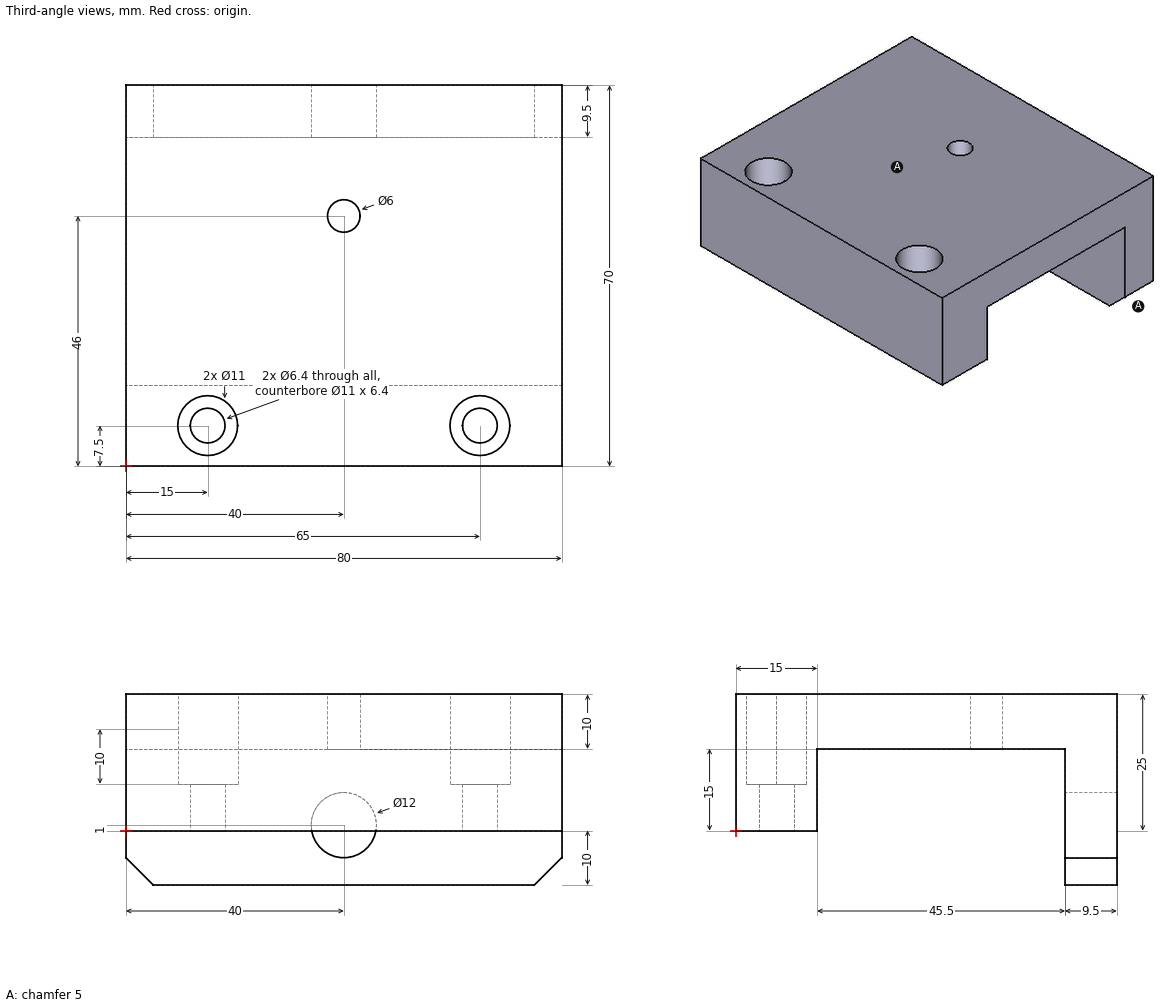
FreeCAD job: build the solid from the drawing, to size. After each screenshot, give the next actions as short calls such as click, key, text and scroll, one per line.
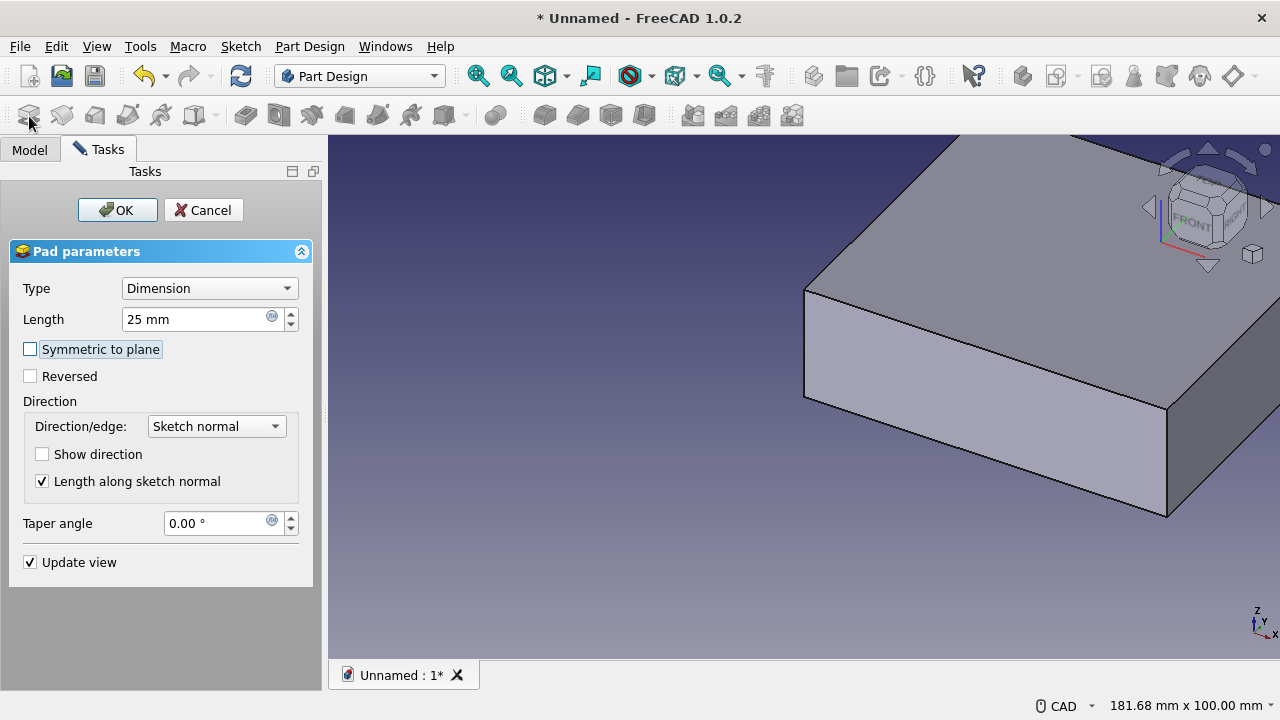
click(118, 210)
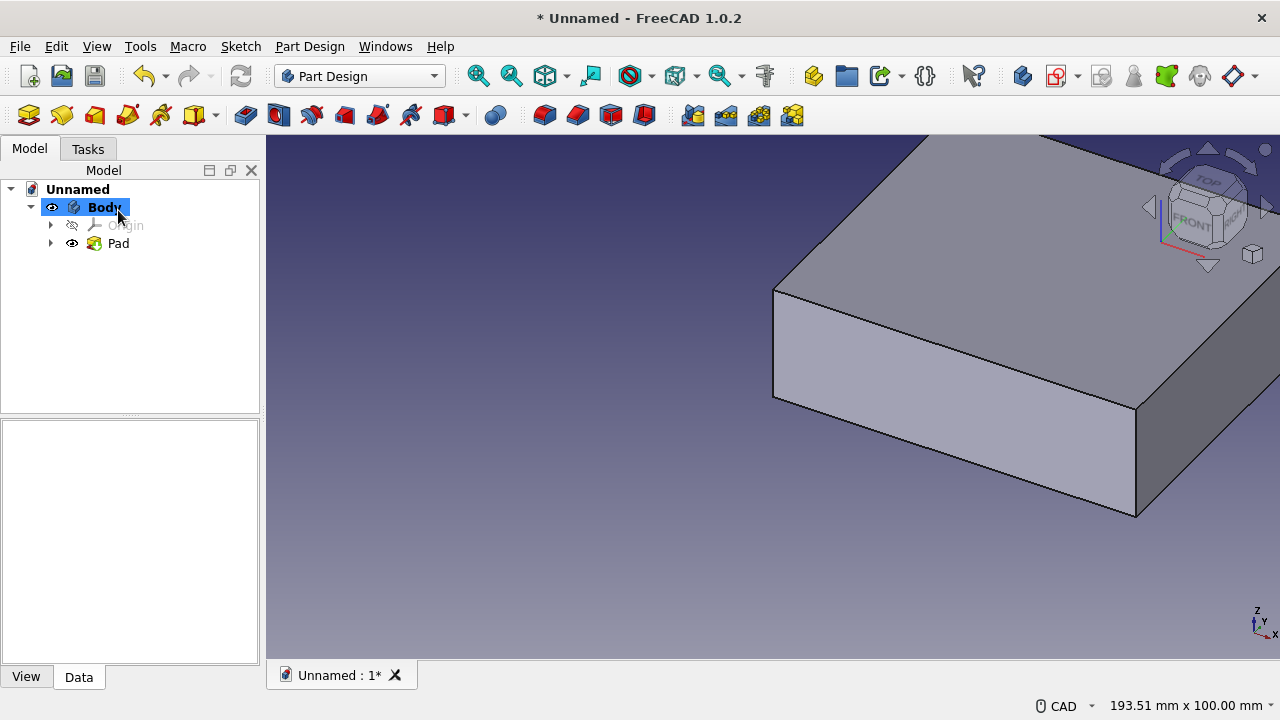
click(479, 76)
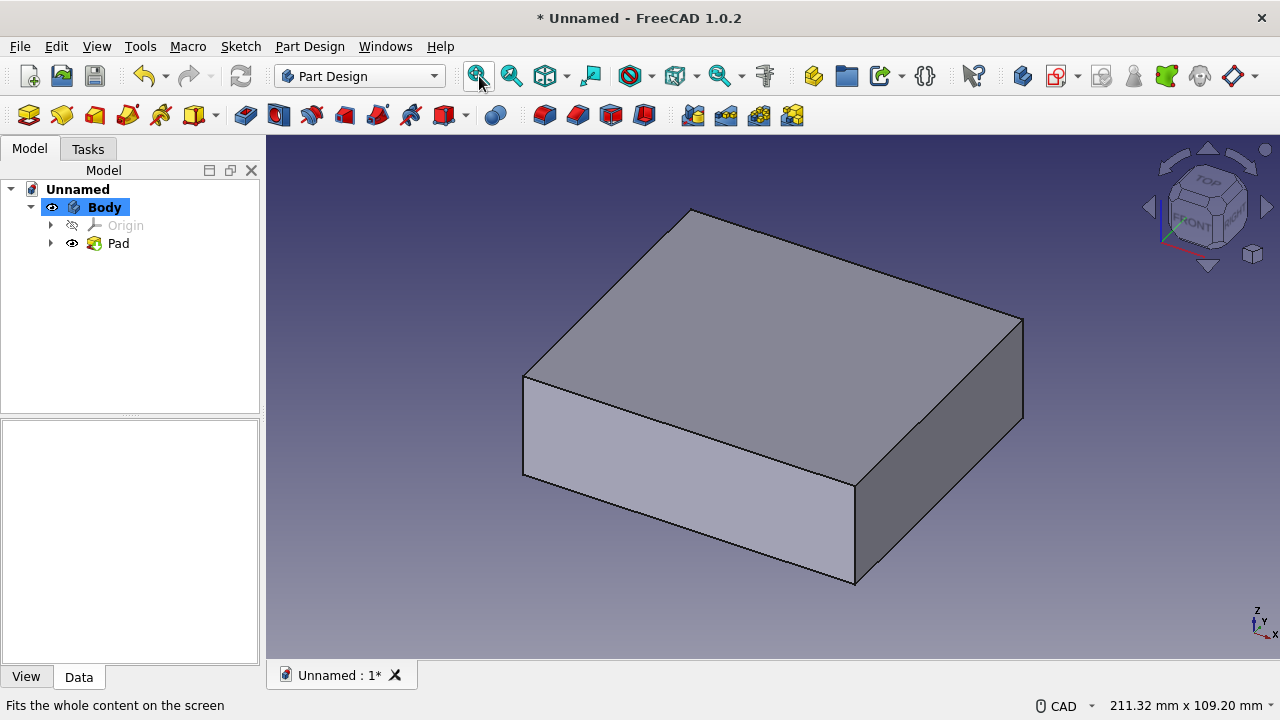
click(987, 403)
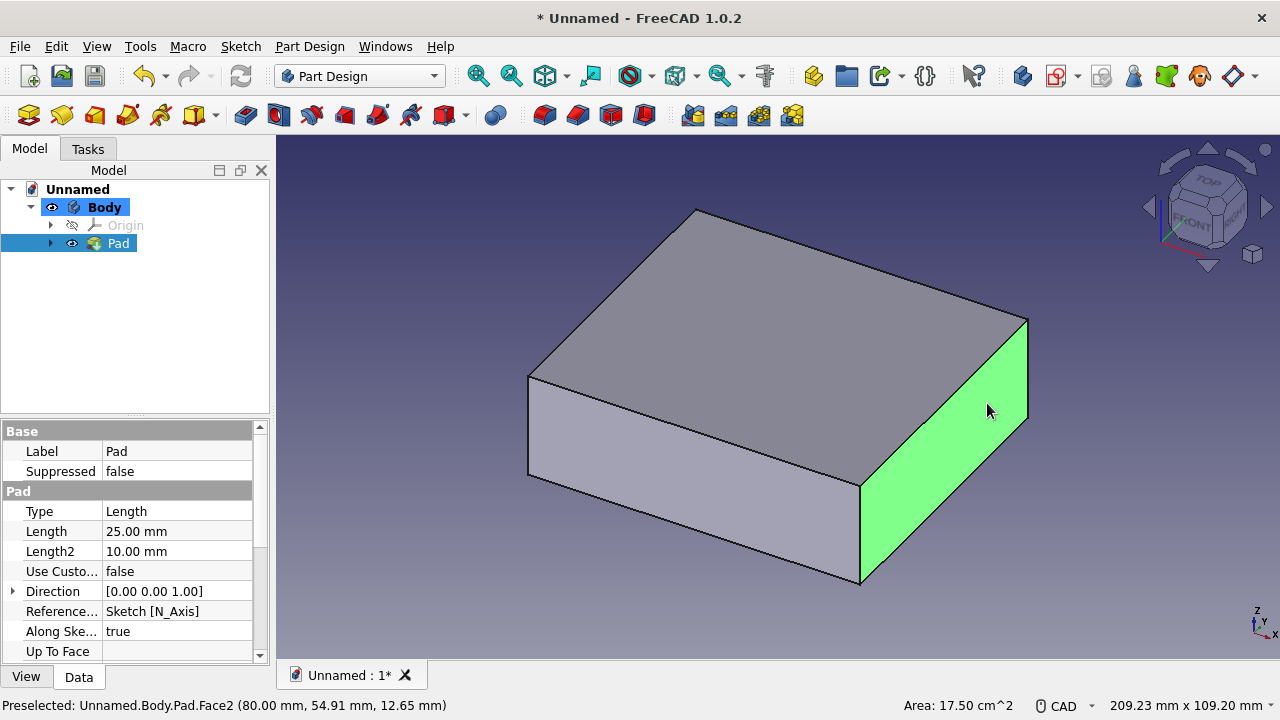
click(1056, 76)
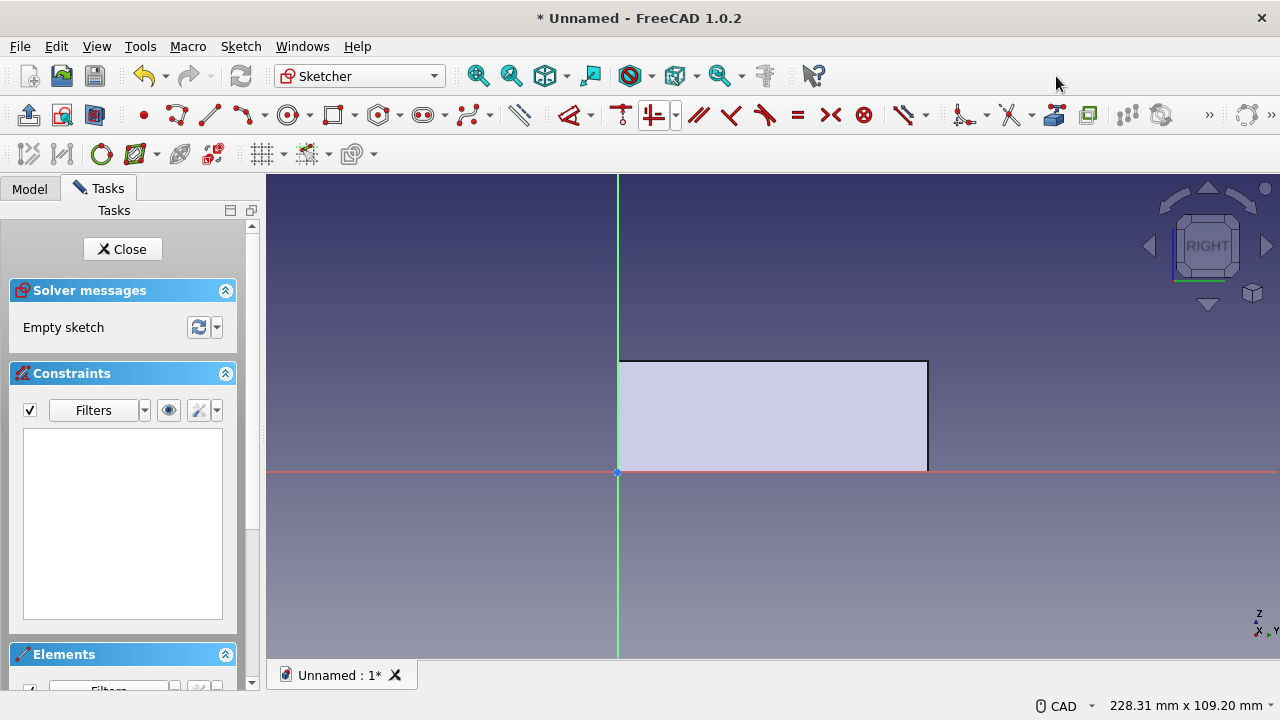
scroll(791, 457, up, 4)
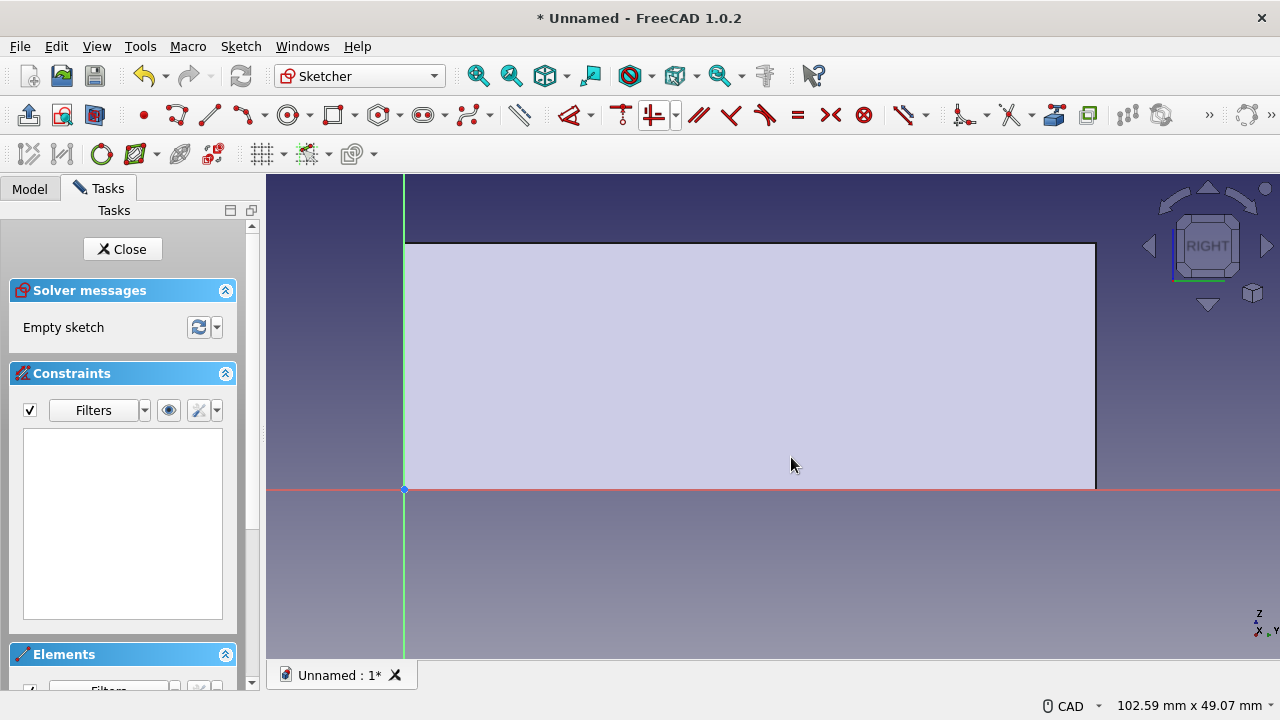
click(332, 116)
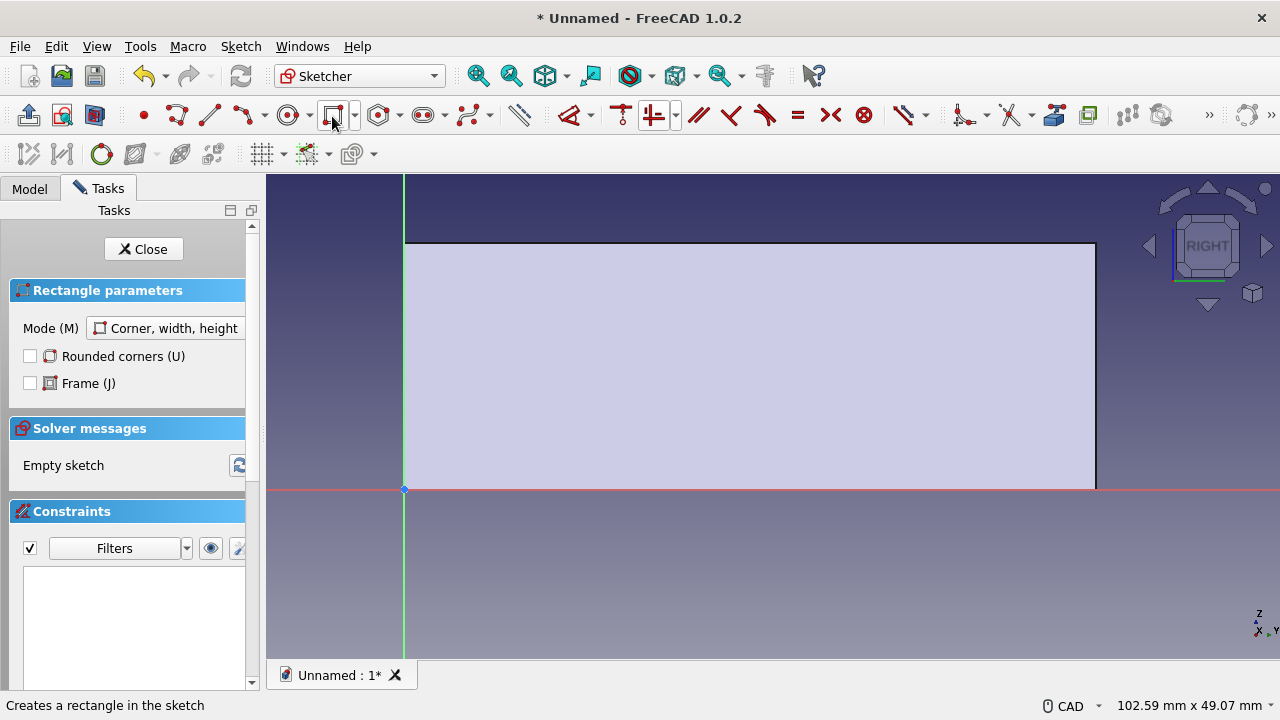
click(553, 341)
click(1002, 490)
key(Escape)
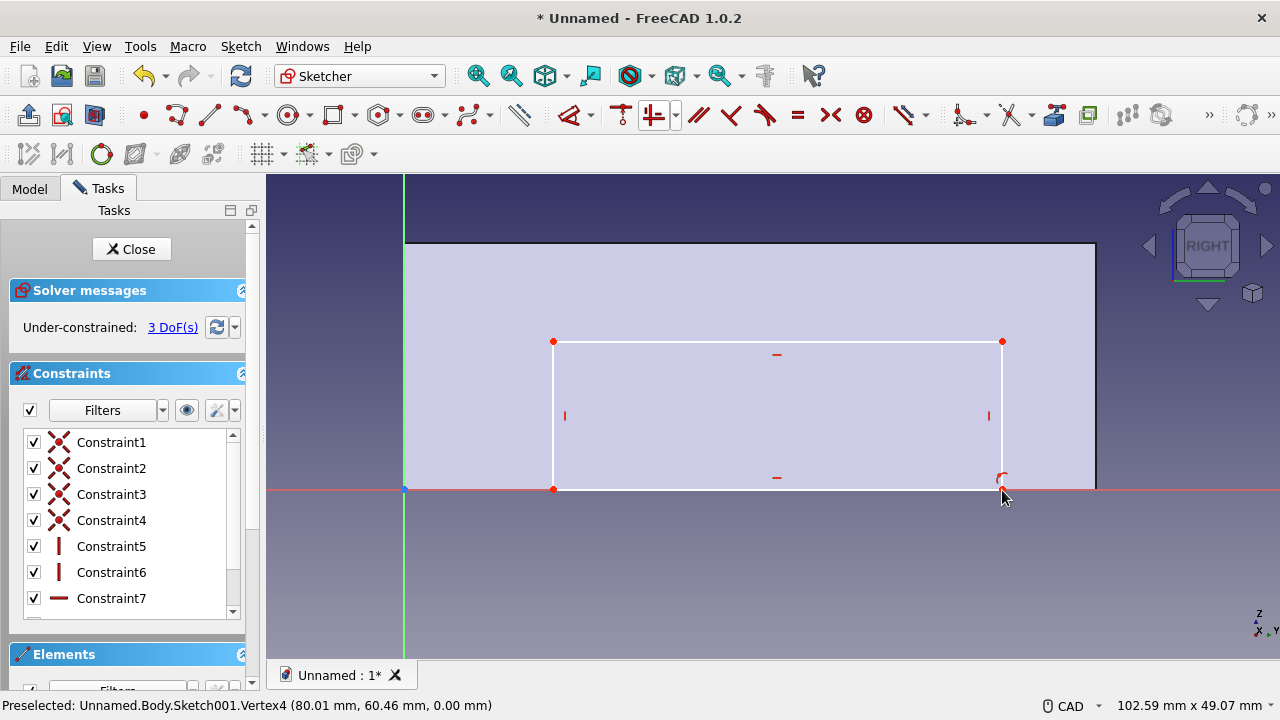
click(553, 386)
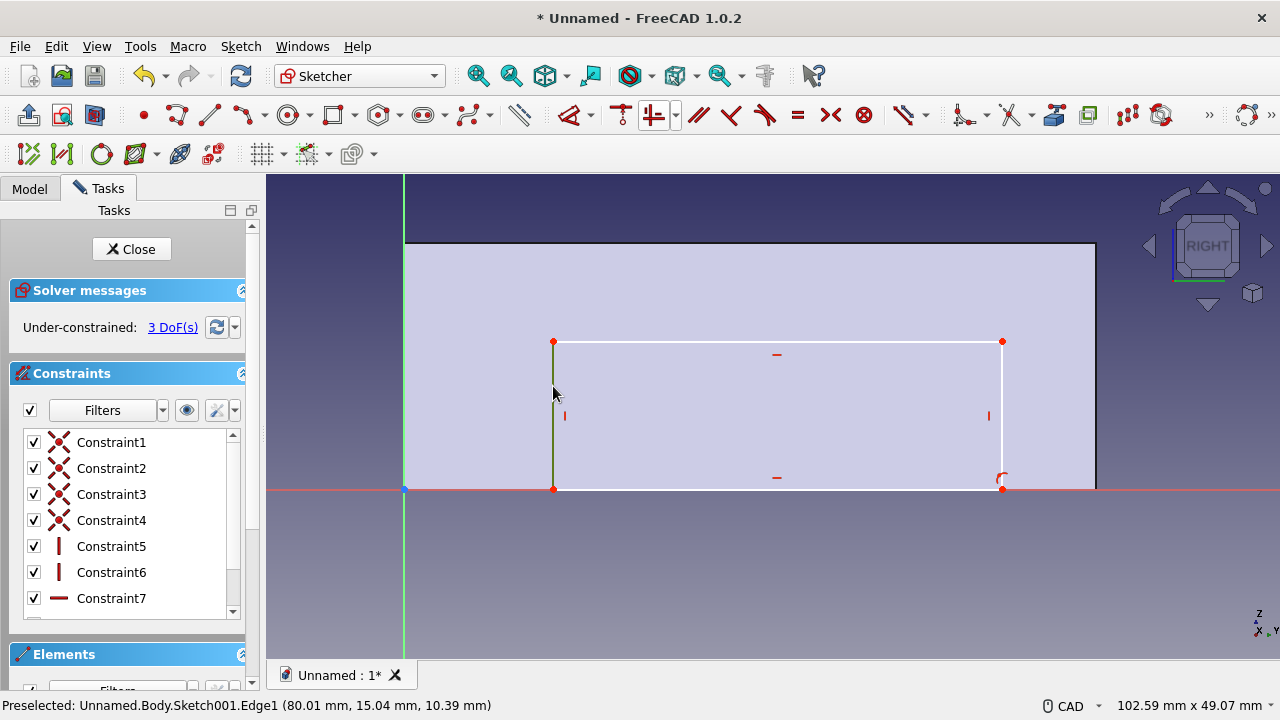
click(590, 116)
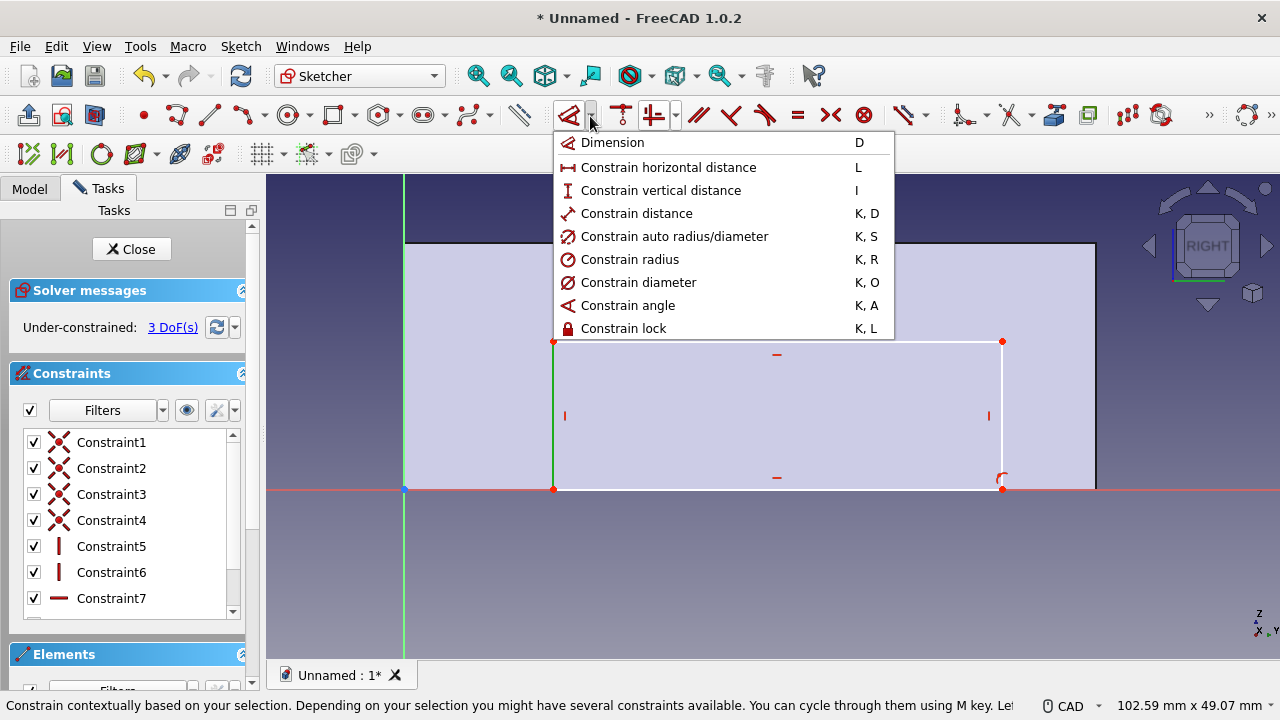
click(724, 190)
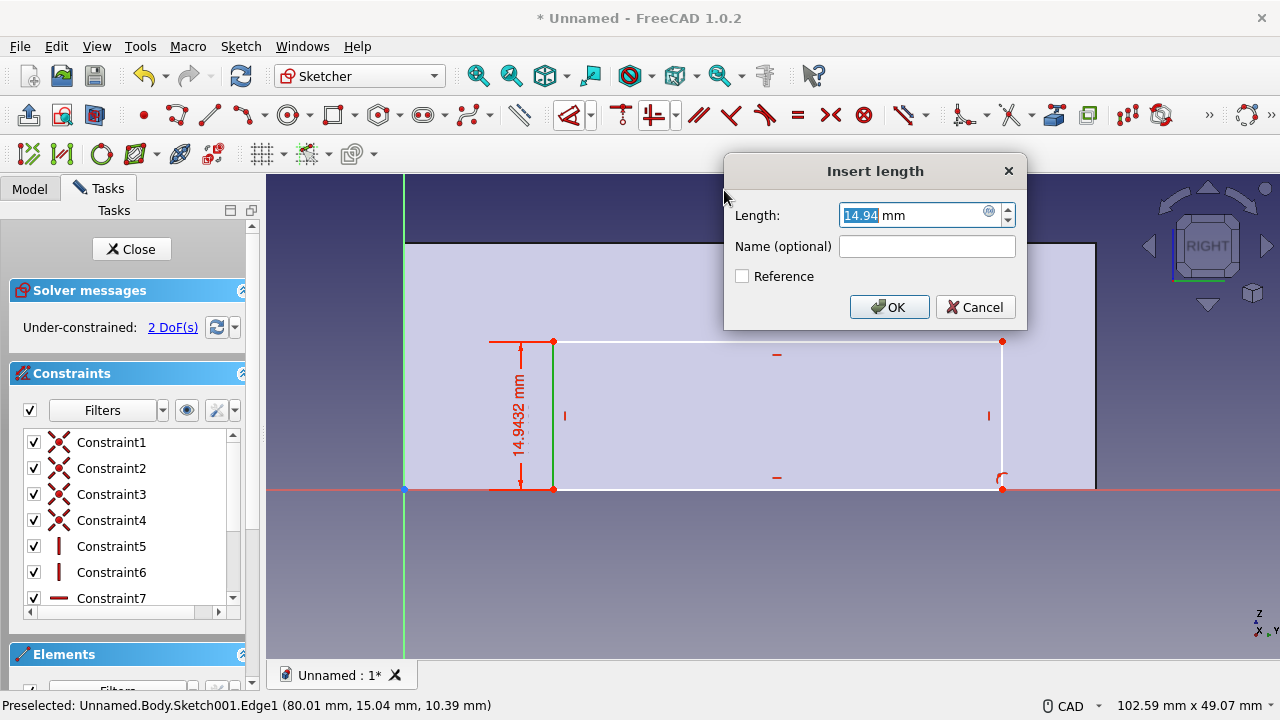
text(15)
key(Return)